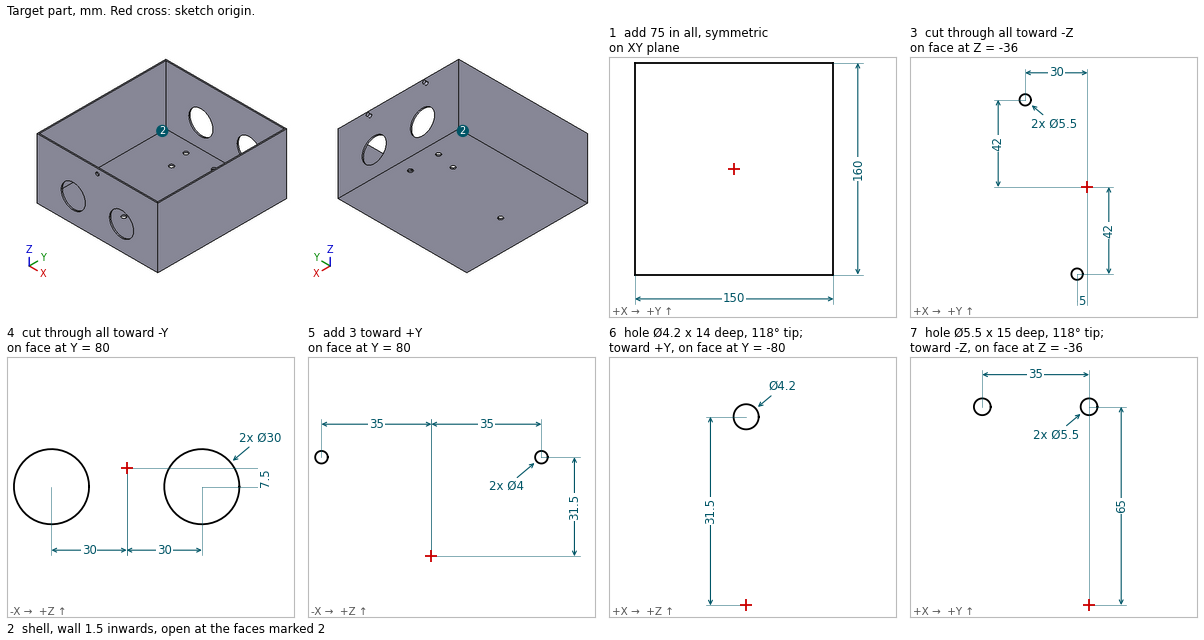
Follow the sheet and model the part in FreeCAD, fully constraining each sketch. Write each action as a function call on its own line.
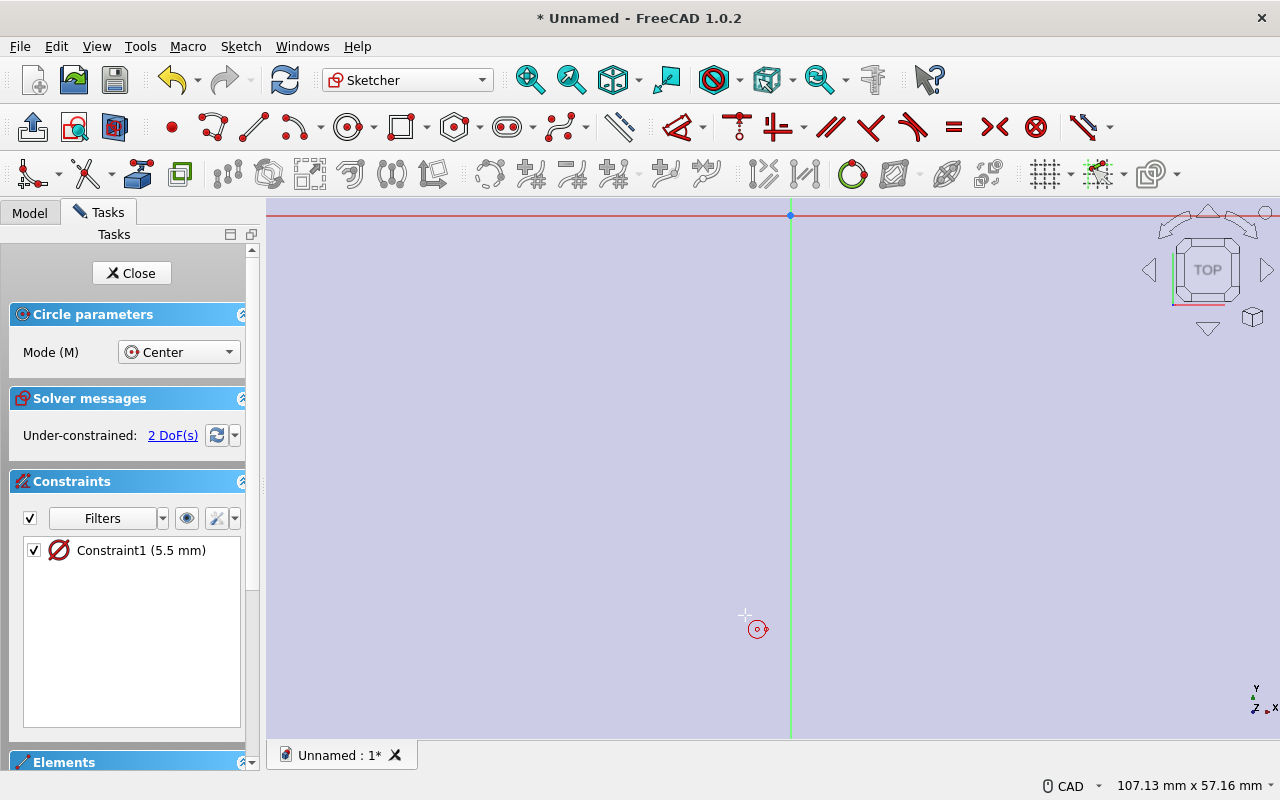
click(743, 613)
move(762, 595)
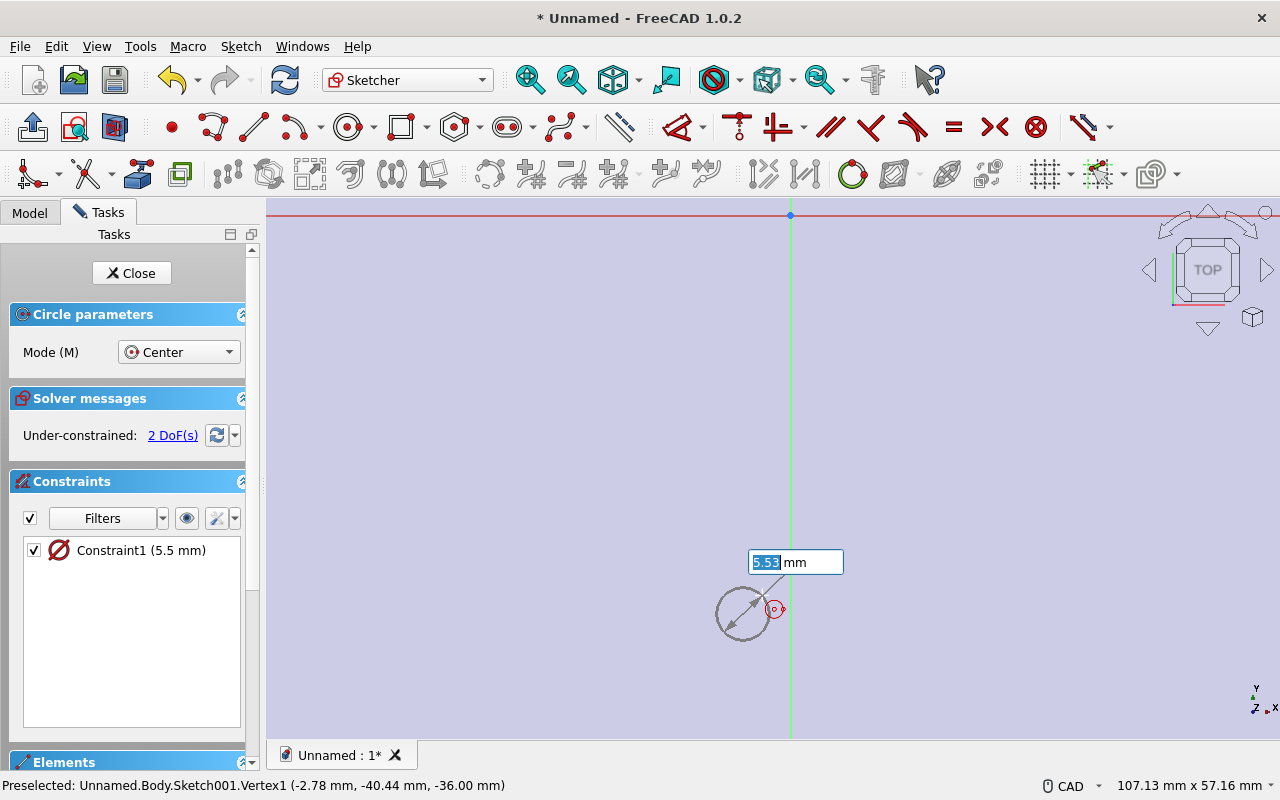
text(5.5)
key(Return)
key(Escape)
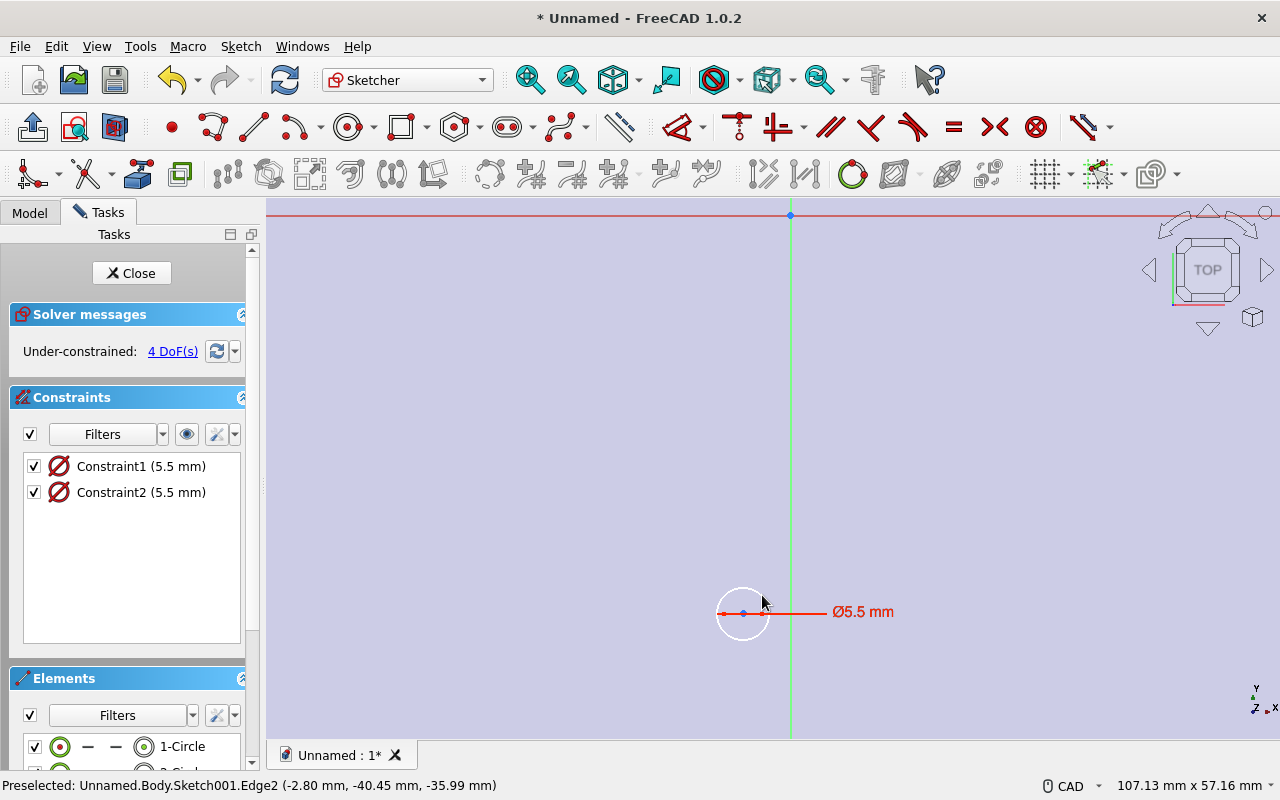
key(d)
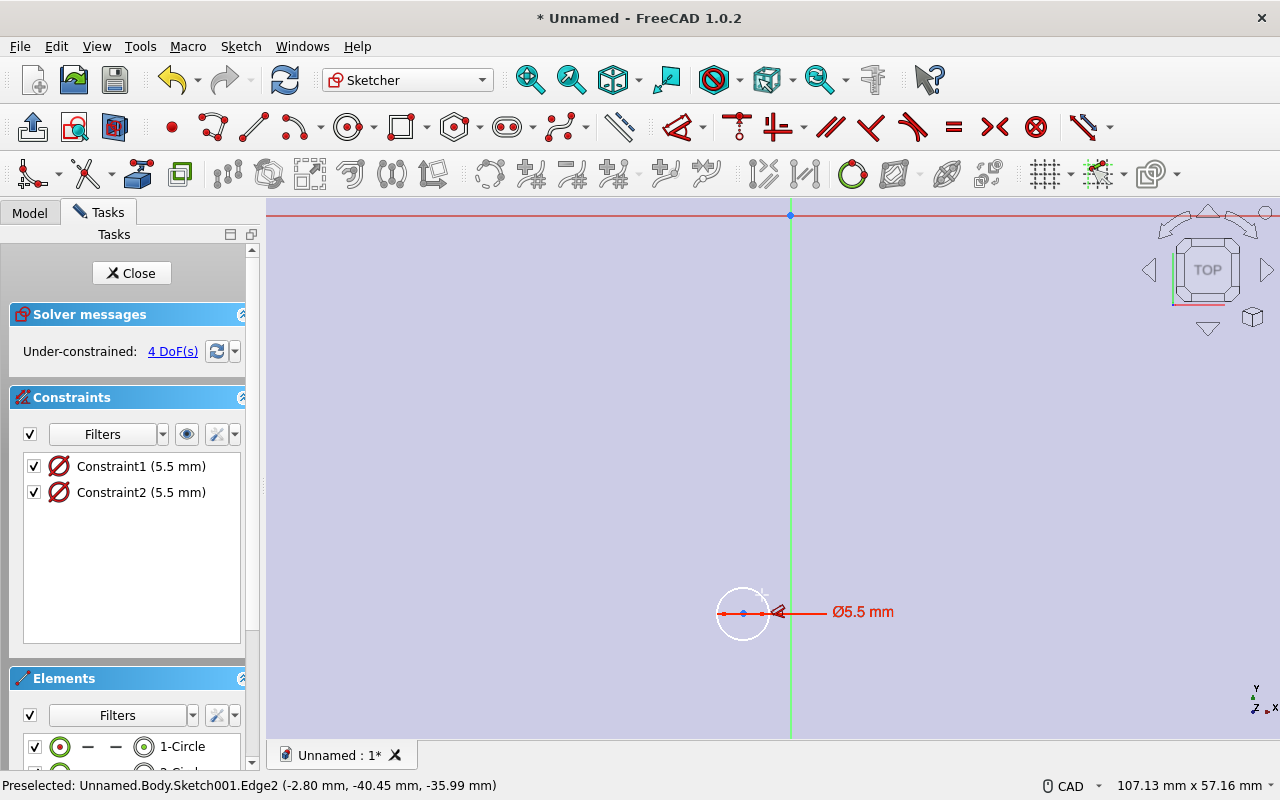
click(743, 614)
click(767, 648)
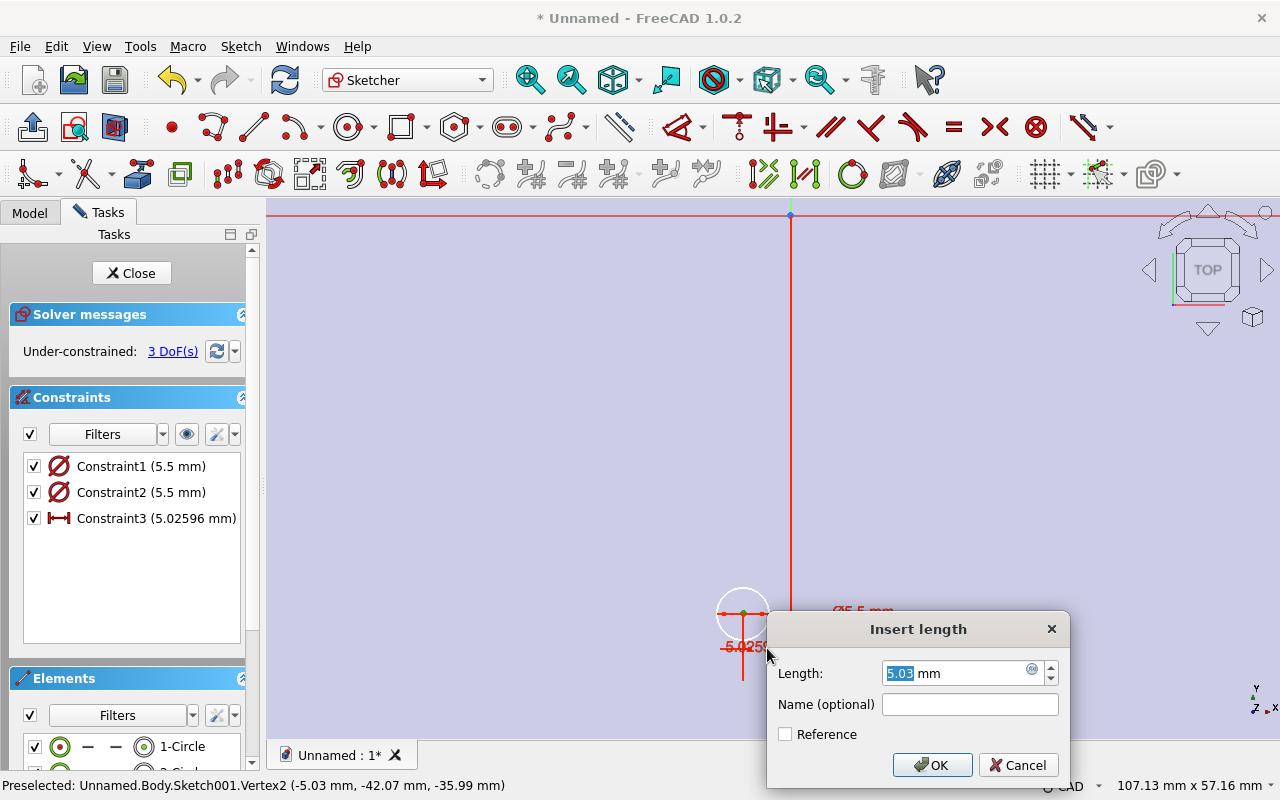
text(5)
key(Return)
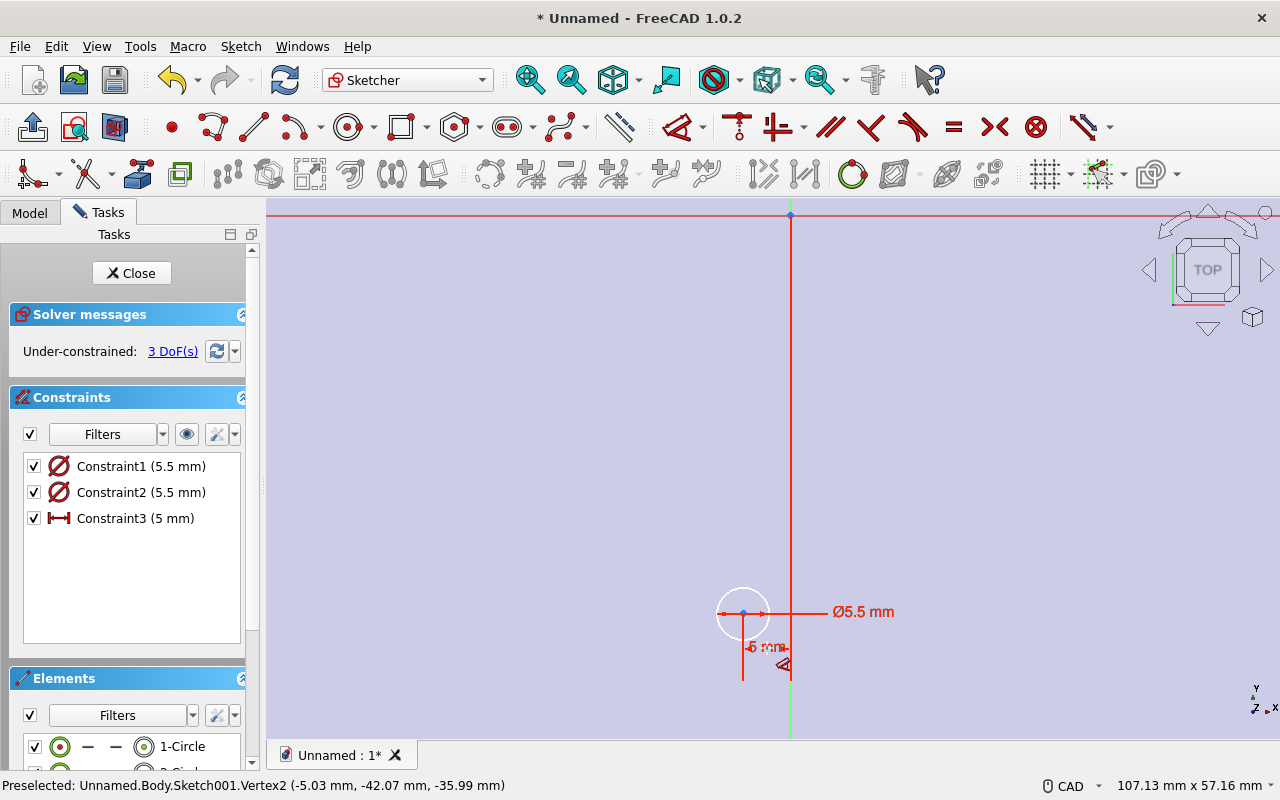
scroll(745, 616, down, 5)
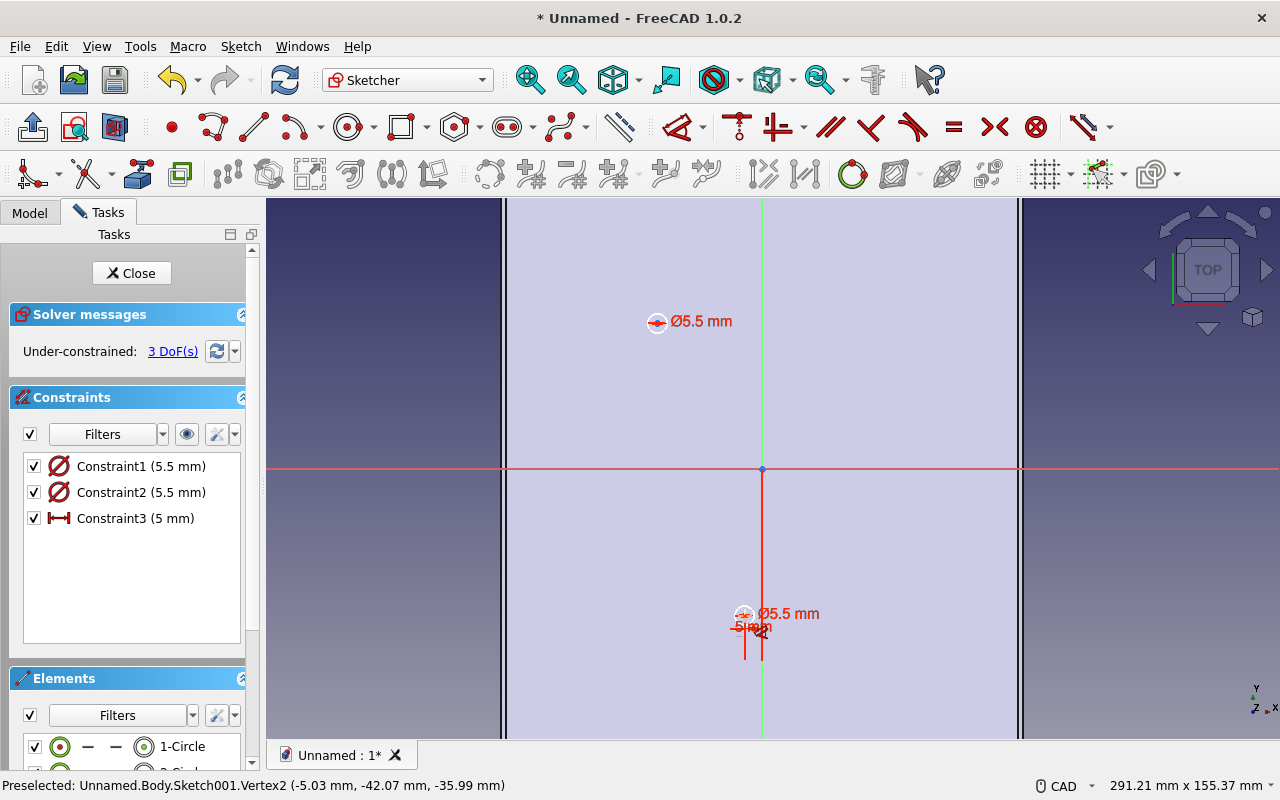
click(658, 323)
click(710, 289)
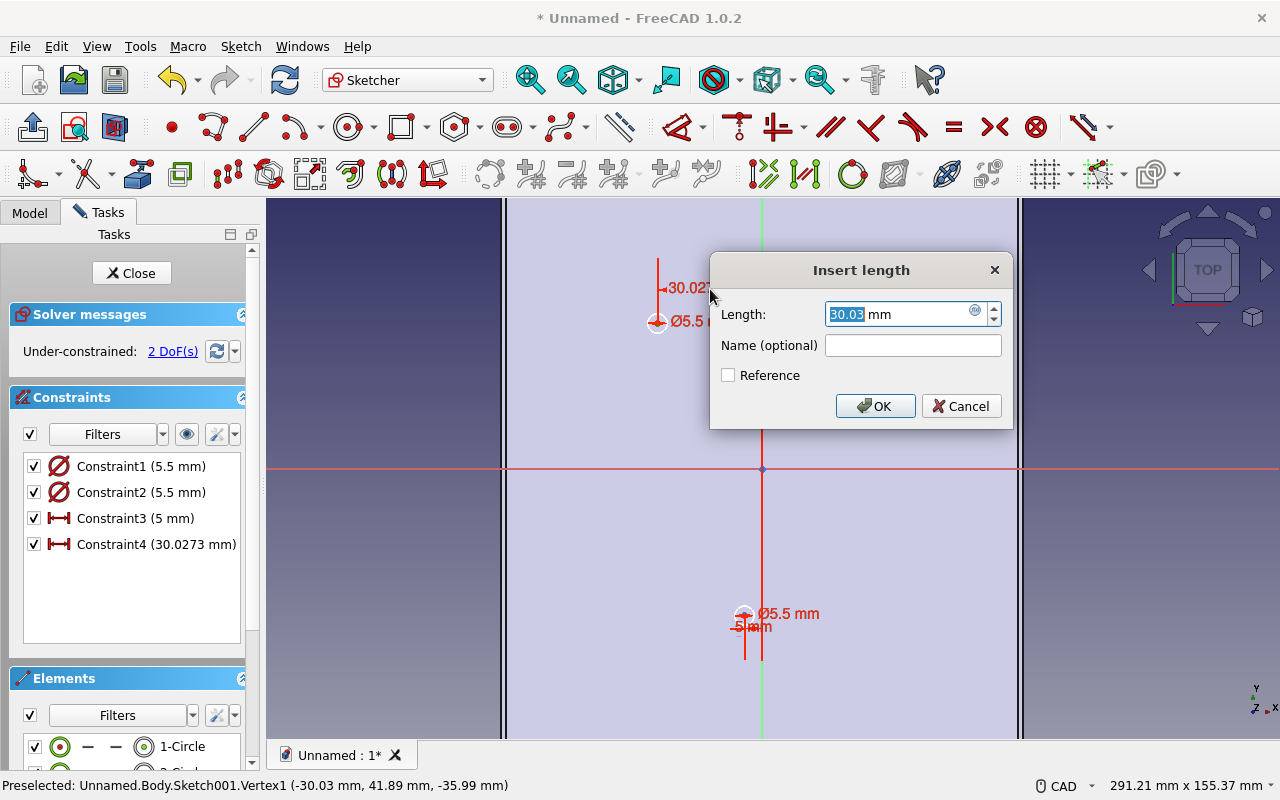
text(30)
key(Return)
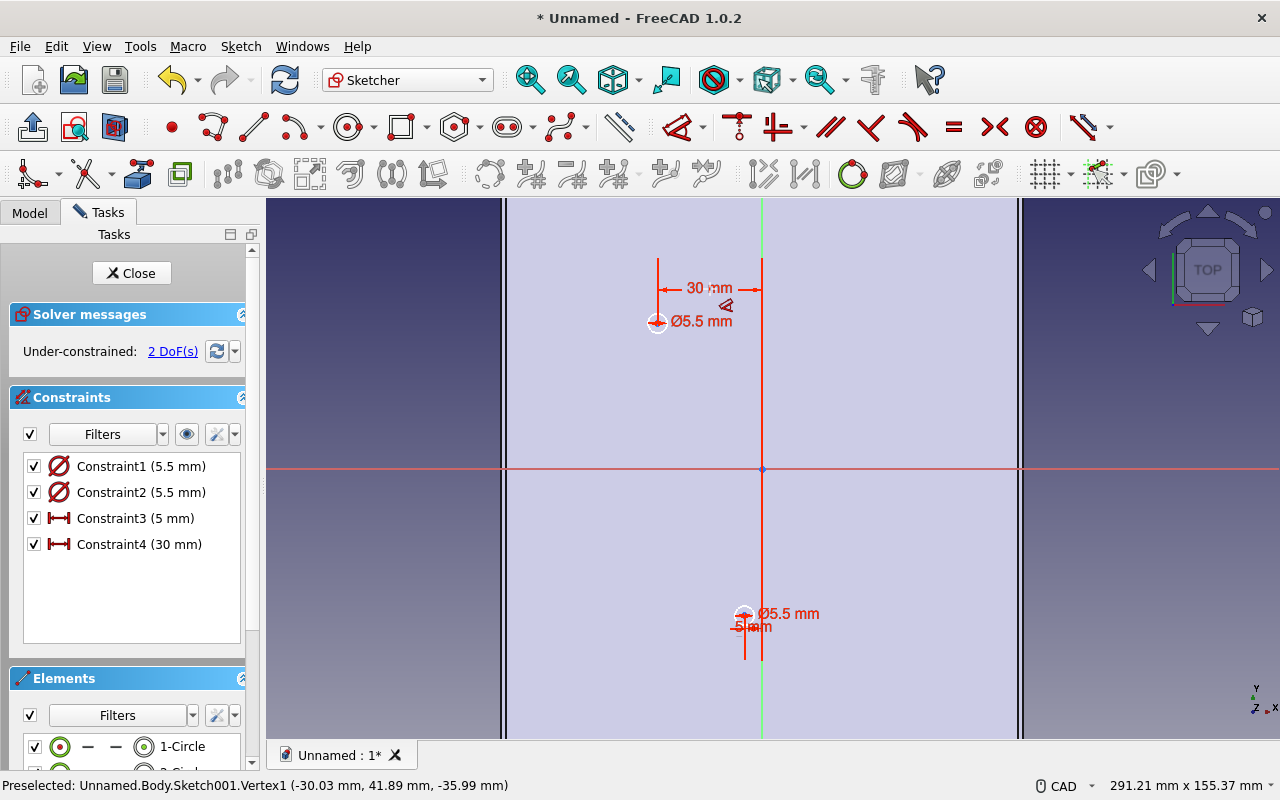
click(658, 323)
click(796, 396)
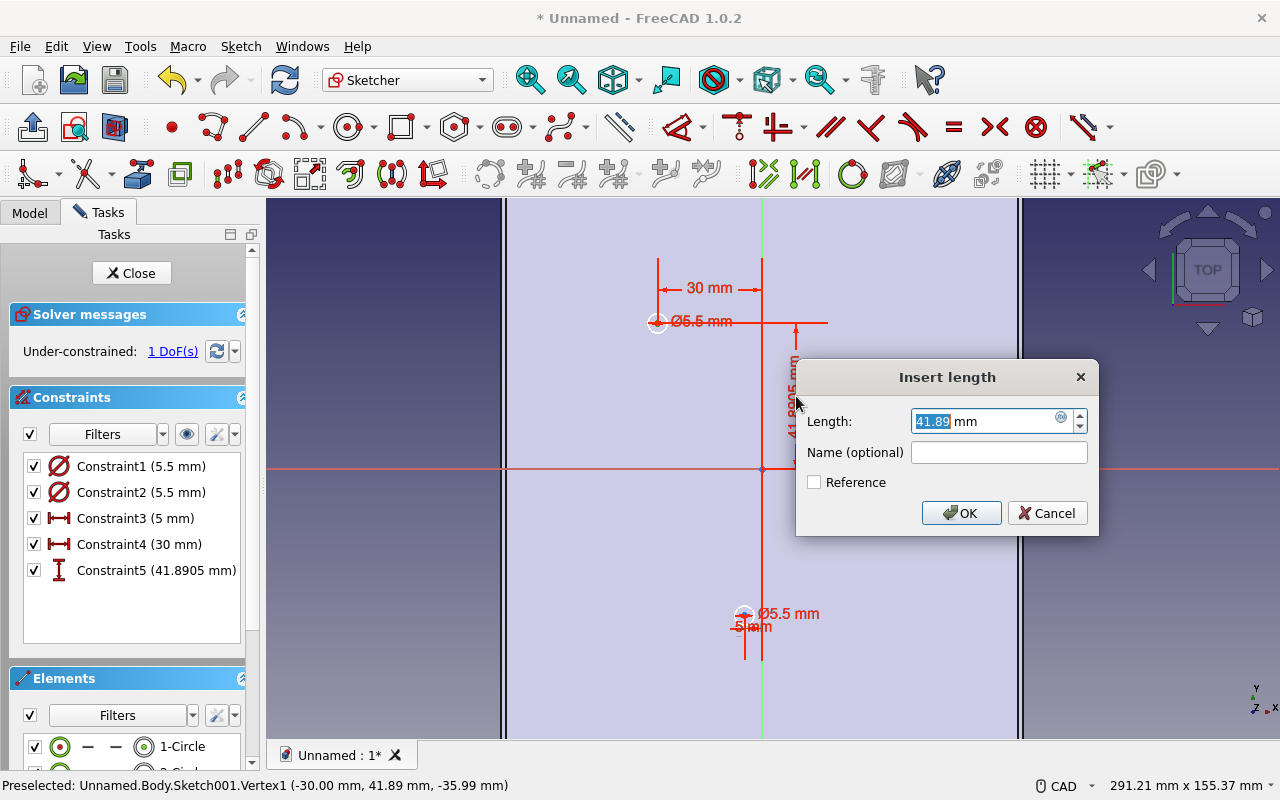
text(42)
key(Return)